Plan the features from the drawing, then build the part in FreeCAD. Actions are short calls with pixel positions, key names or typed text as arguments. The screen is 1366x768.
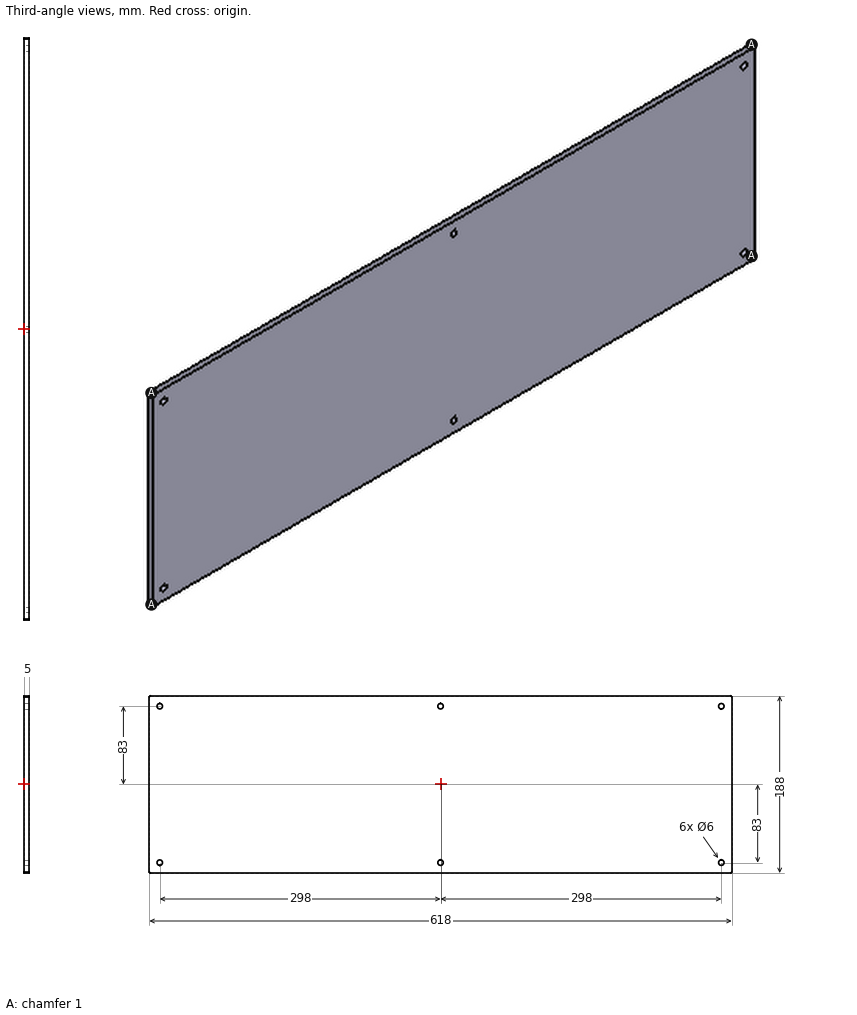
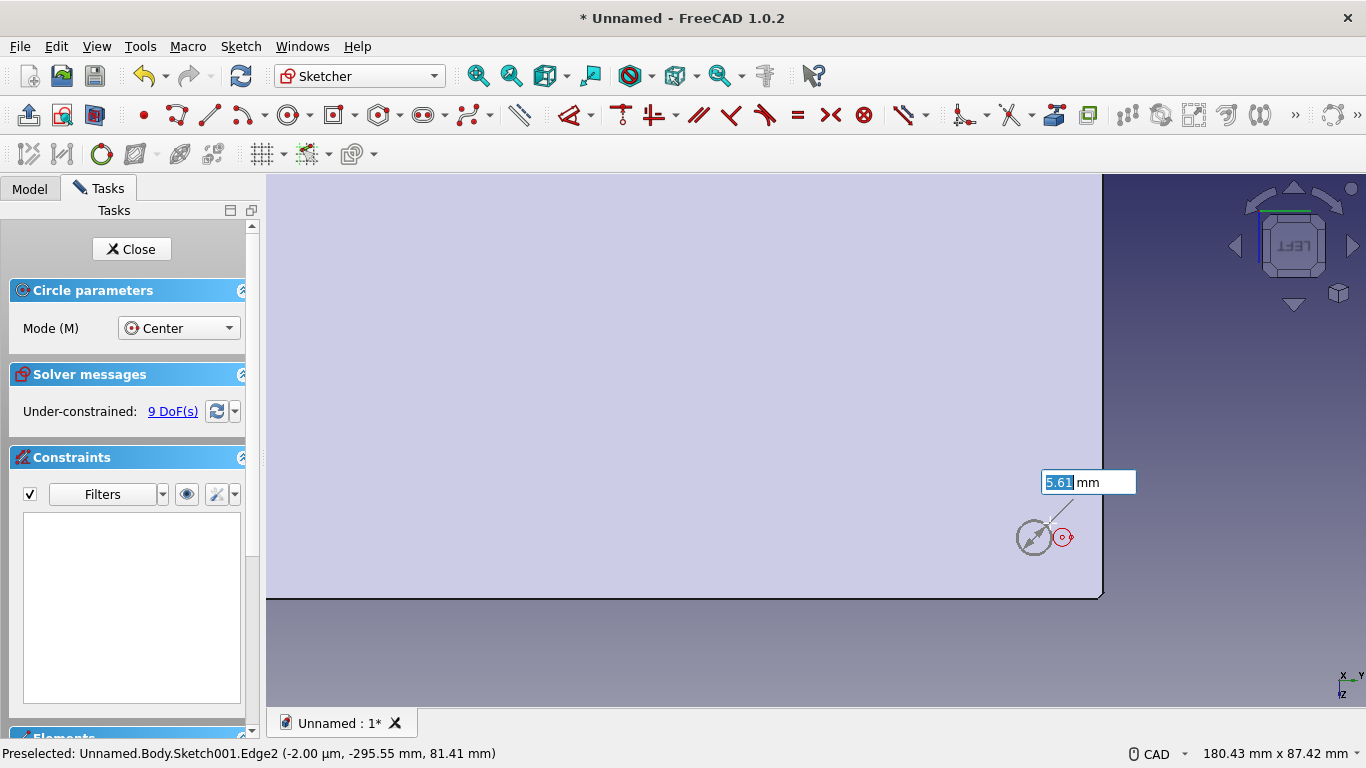
click(1049, 519)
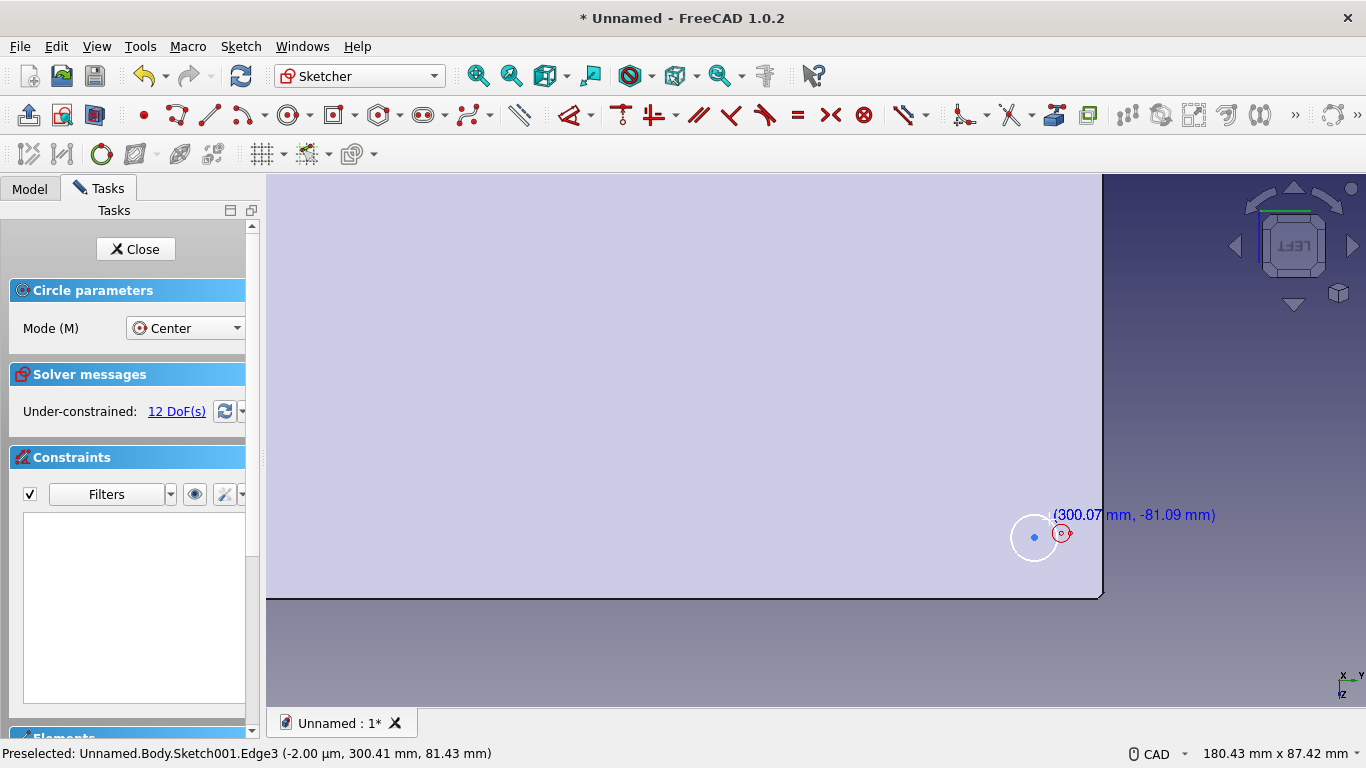
scroll(1050, 523, down, 9)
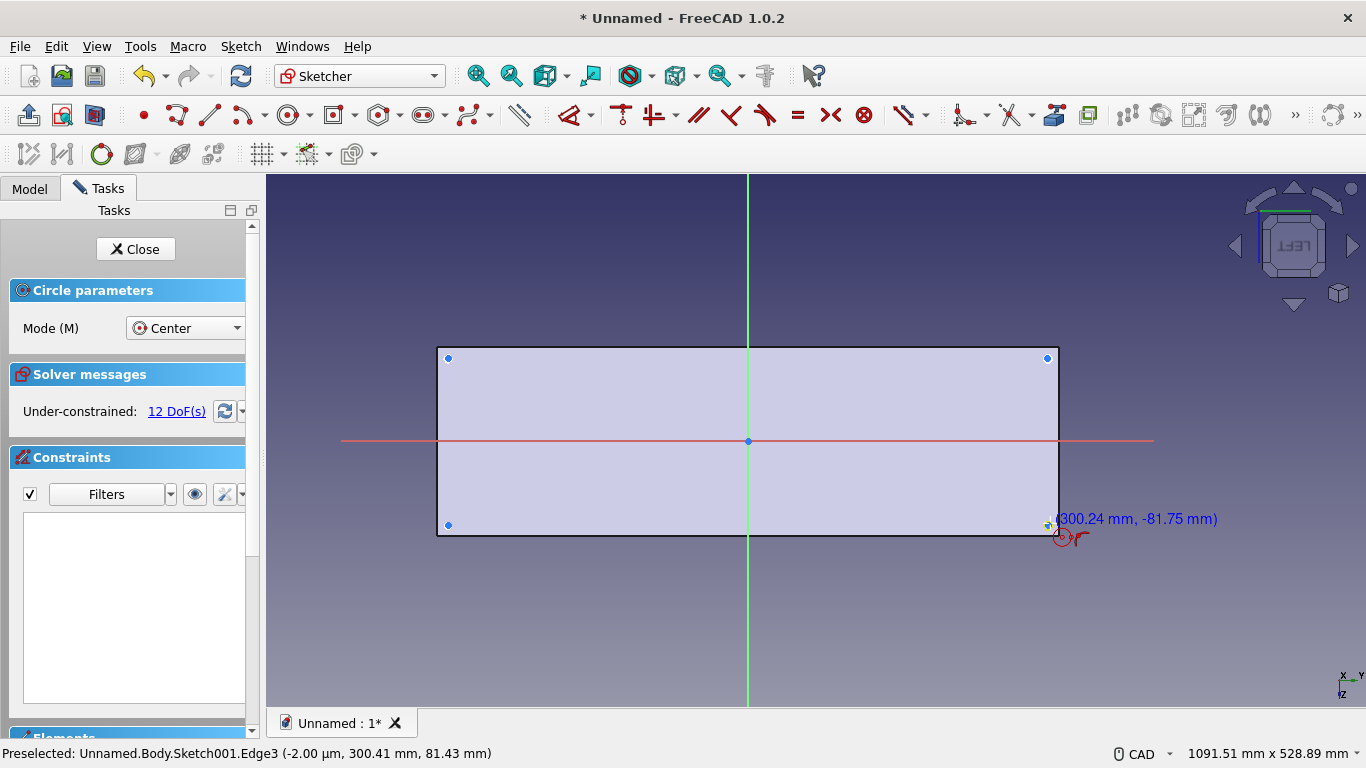
scroll(748, 525, up, 11)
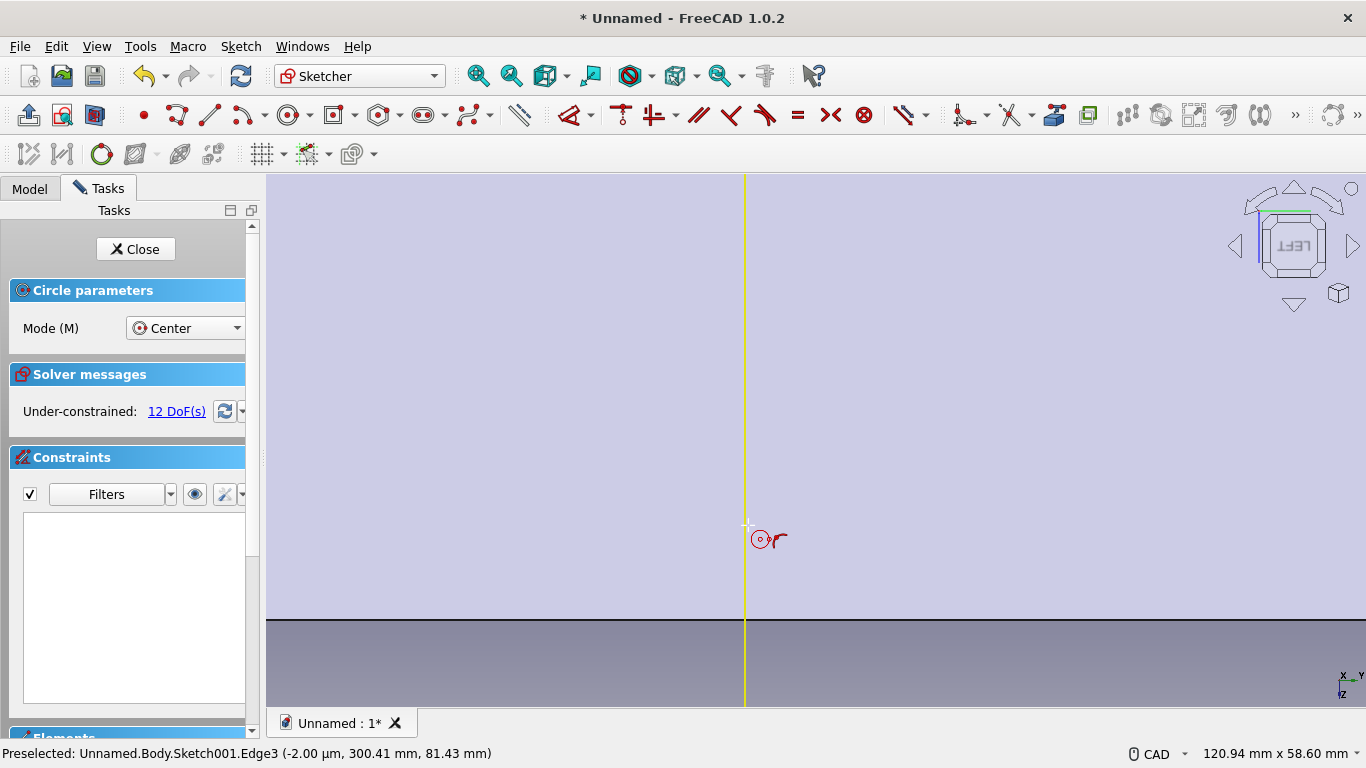
scroll(748, 525, down, 11)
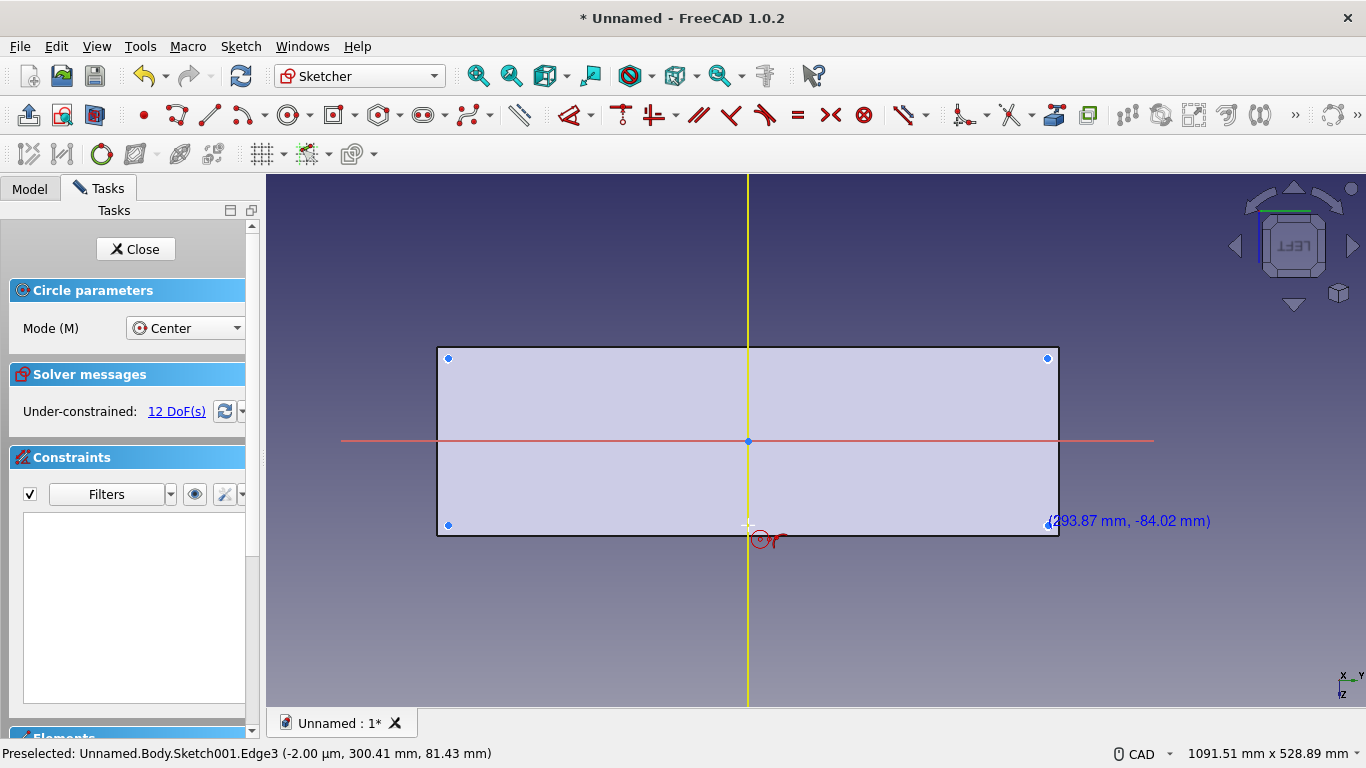
click(748, 525)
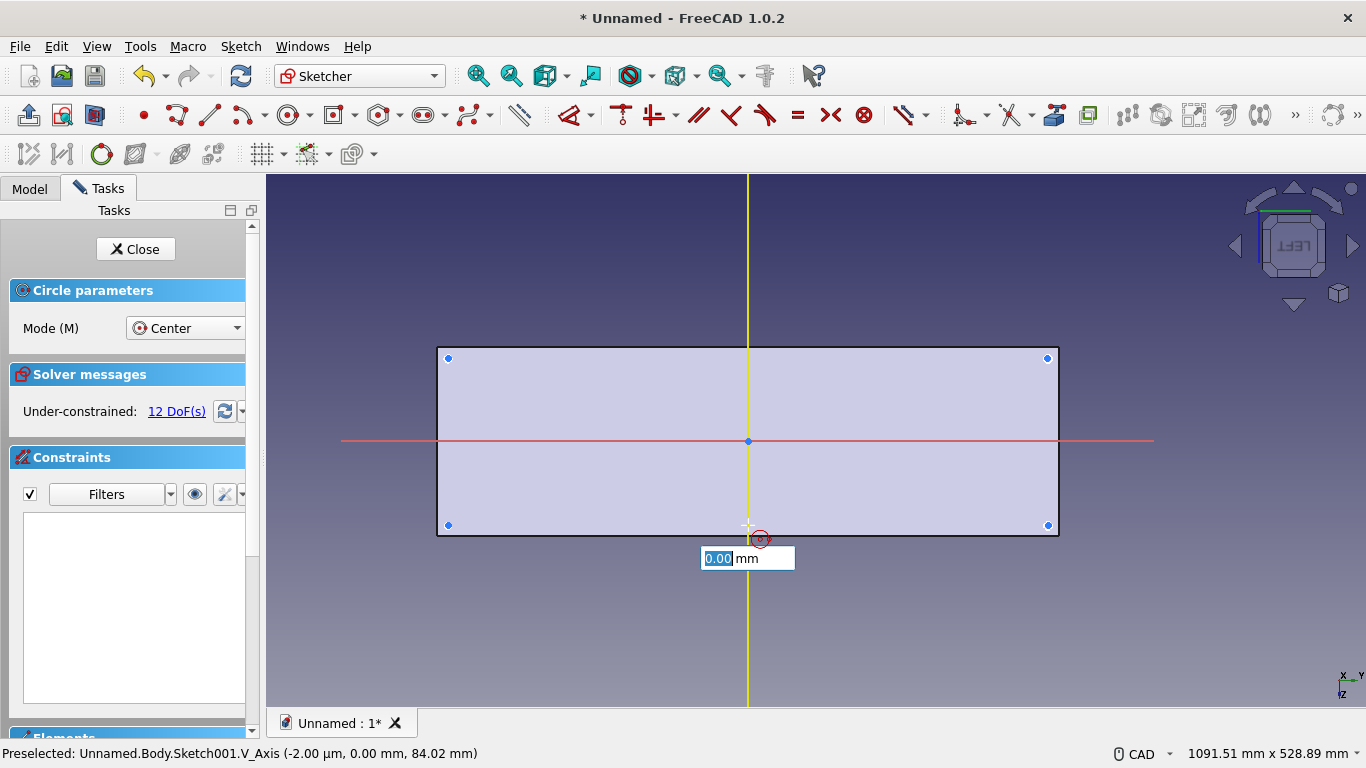
scroll(751, 524, up, 9)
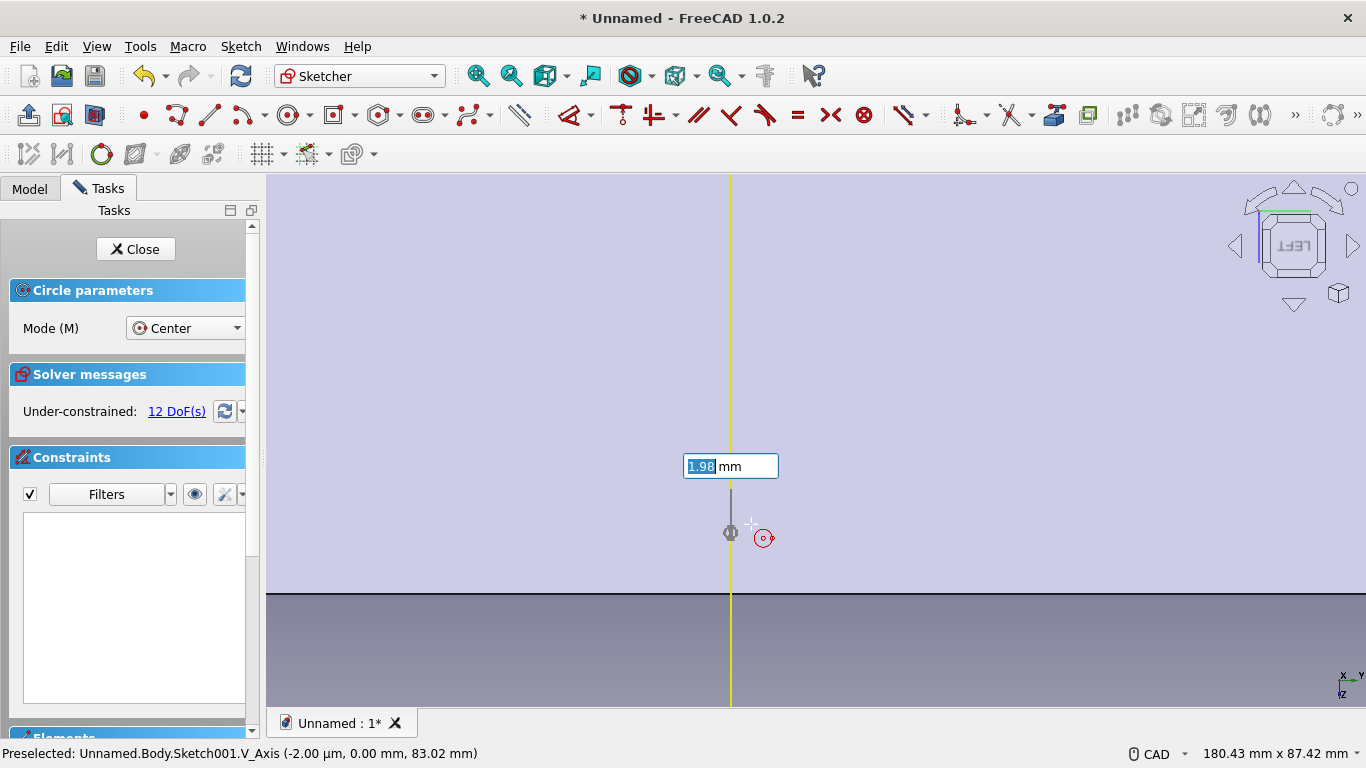
click(748, 520)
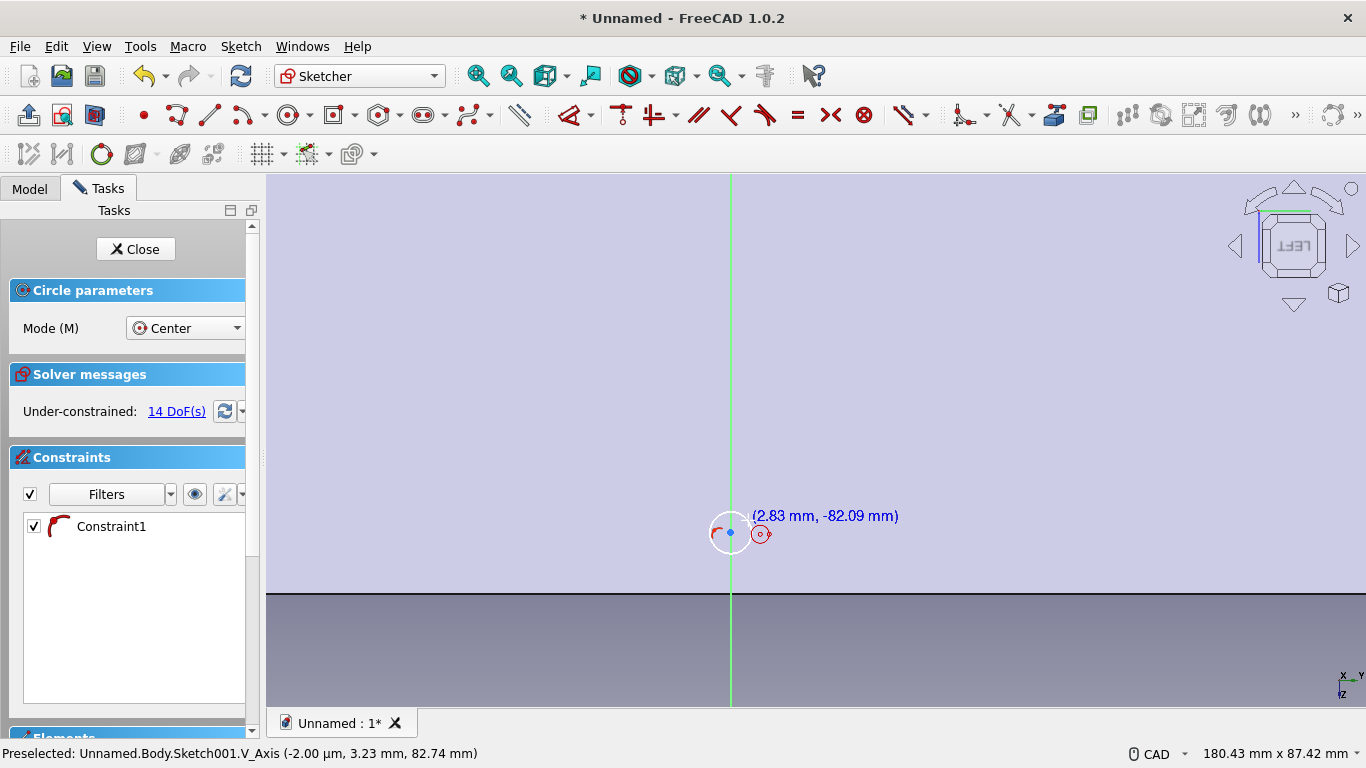
scroll(751, 524, down, 9)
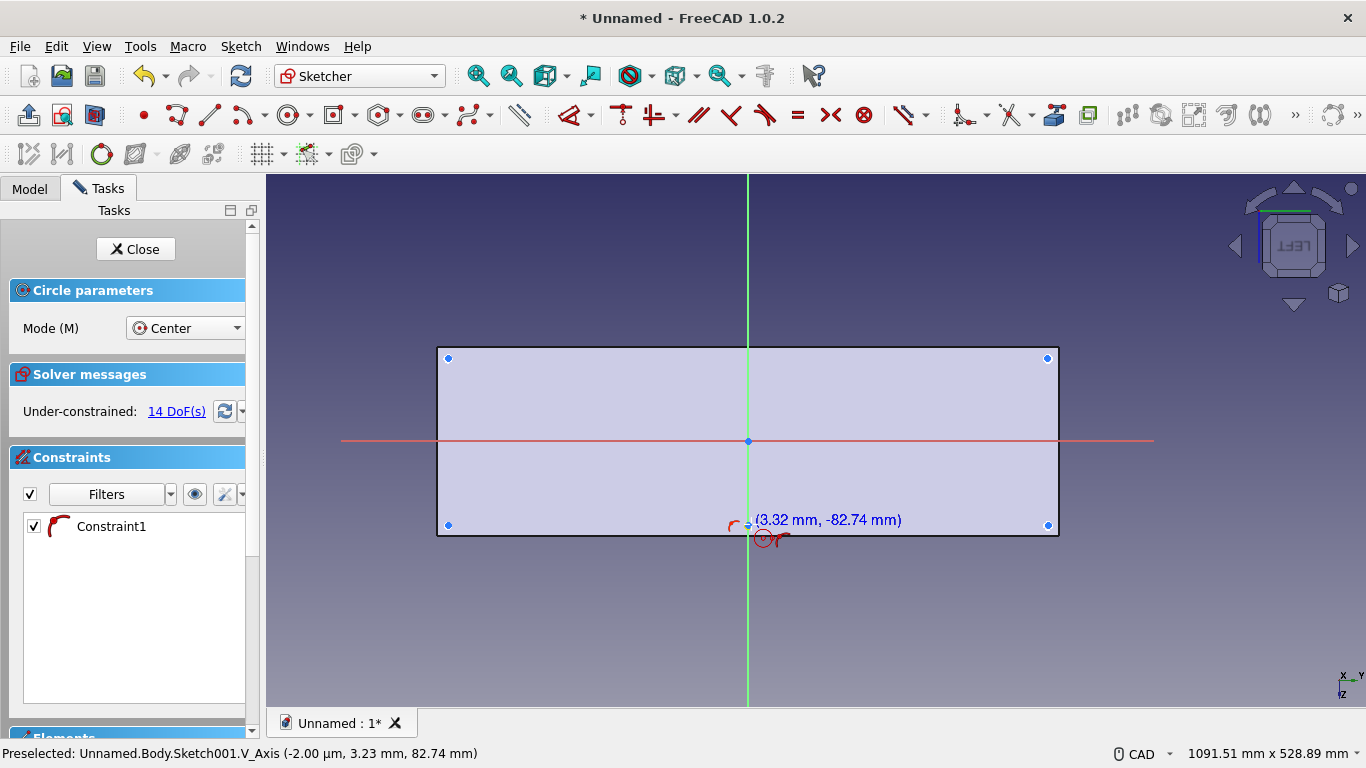
scroll(748, 358, up, 11)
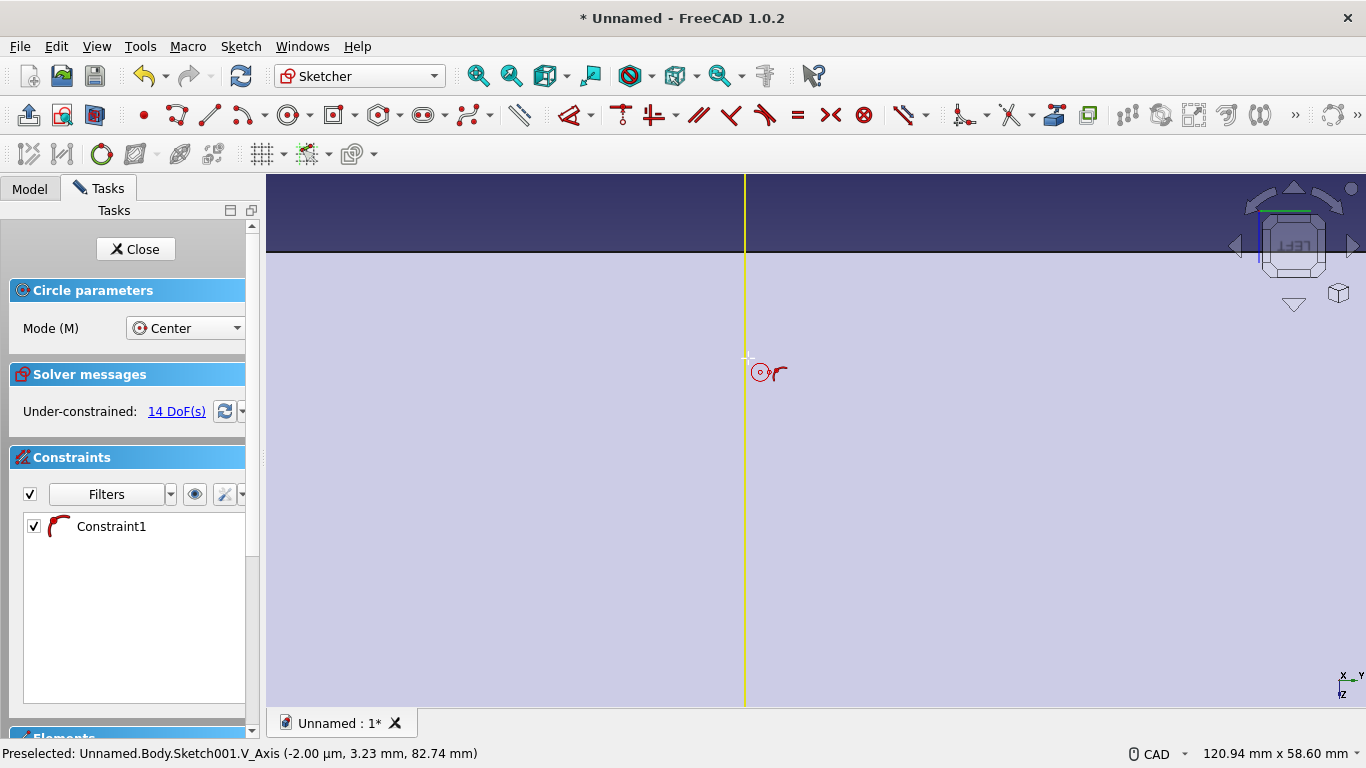
scroll(748, 357, down, 11)